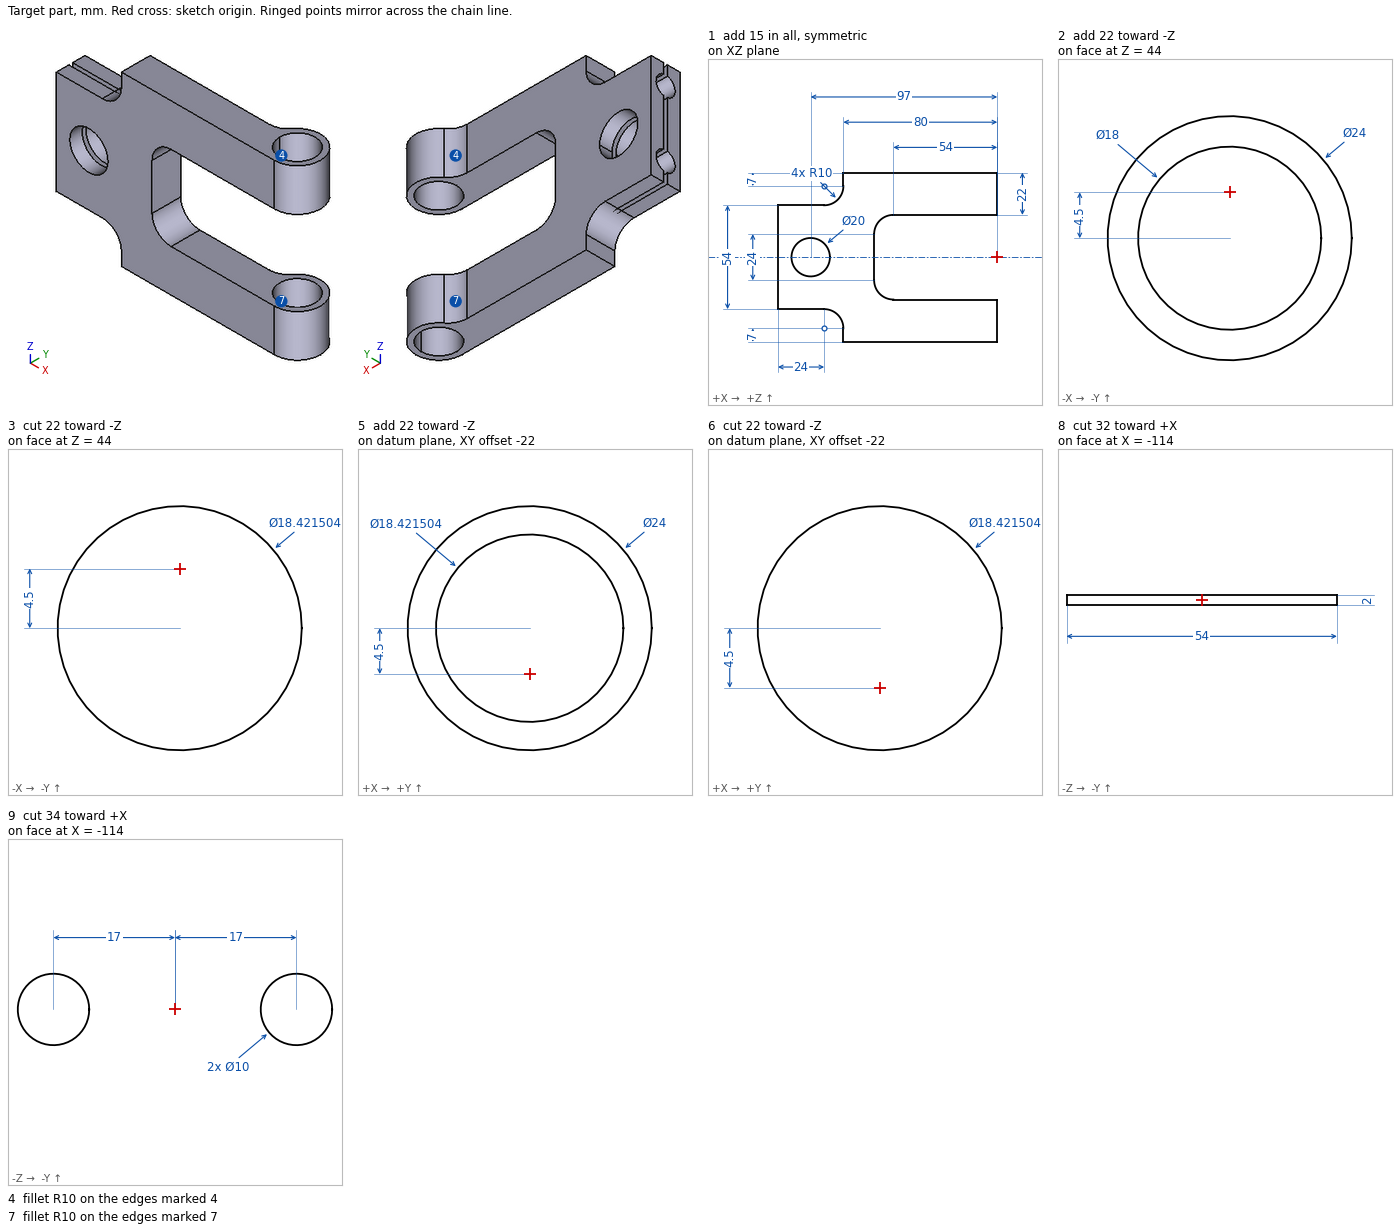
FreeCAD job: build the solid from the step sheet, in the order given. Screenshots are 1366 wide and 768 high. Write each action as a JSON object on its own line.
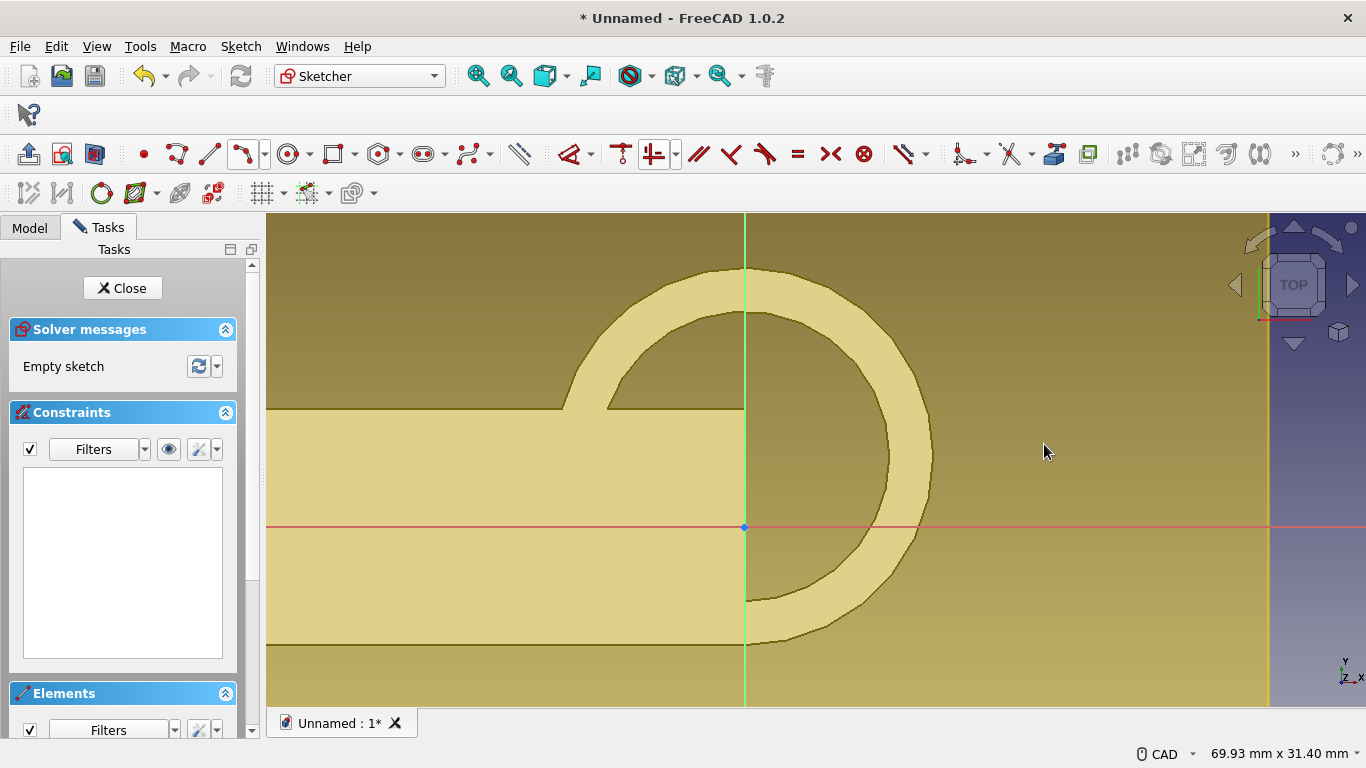
{"action": "left_click", "coordinate": [288, 154]}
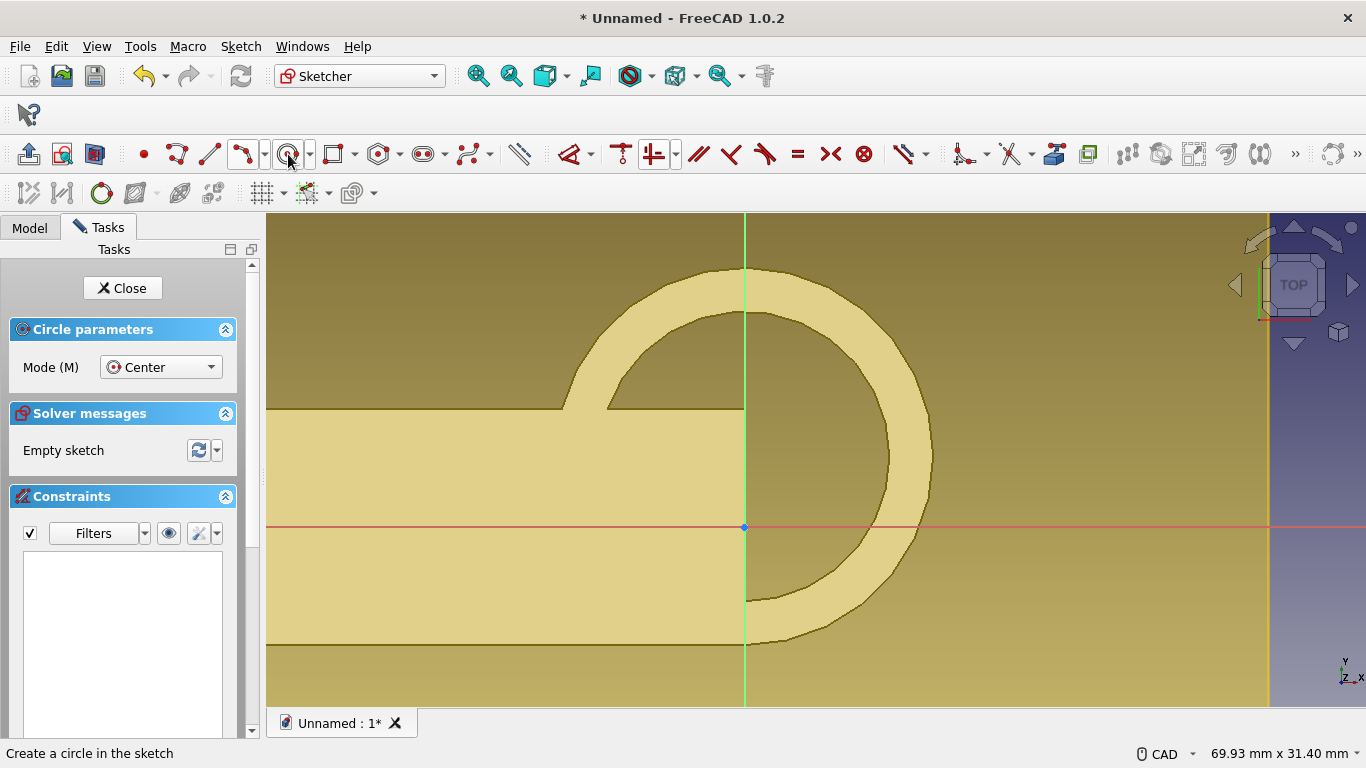
{"action": "left_click", "coordinate": [745, 456]}
{"action": "left_click", "coordinate": [847, 354]}
{"action": "key", "text": "Escape"}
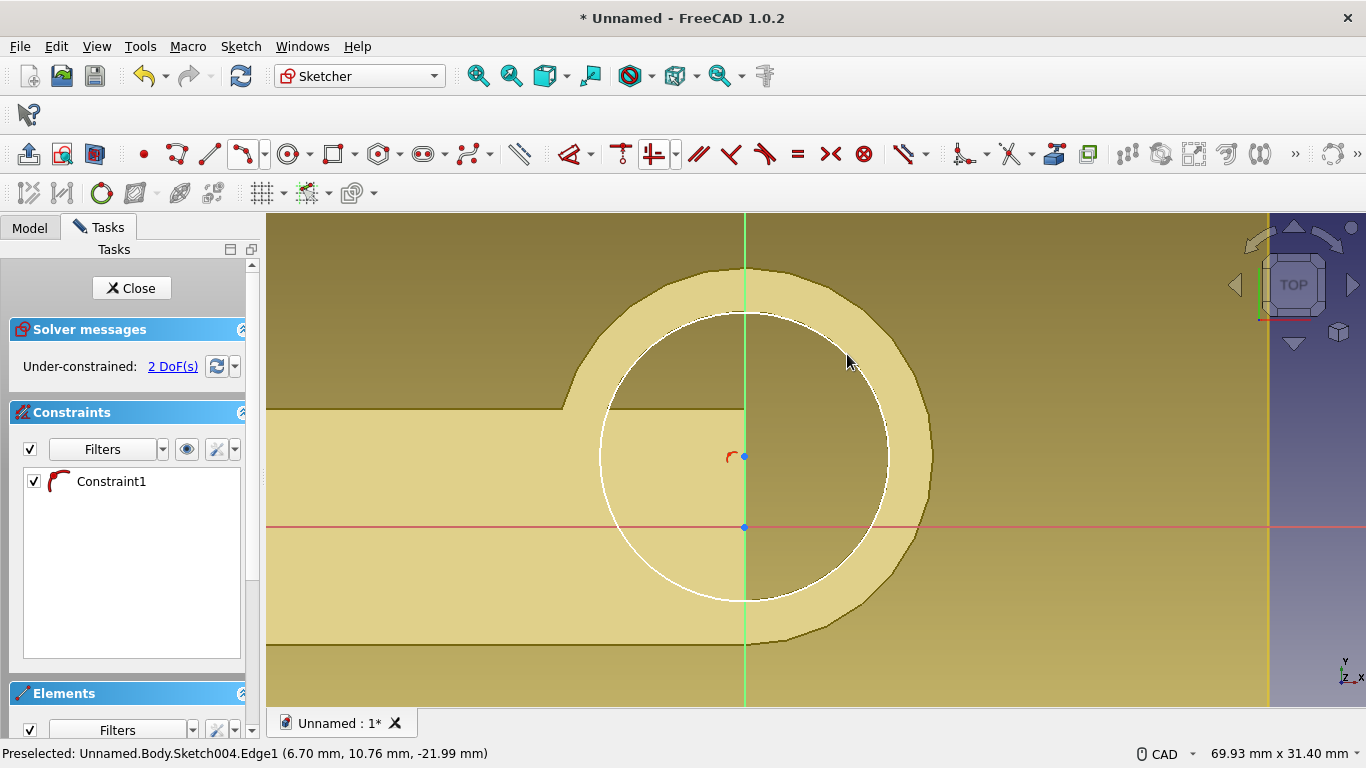
{"action": "left_click", "coordinate": [568, 154]}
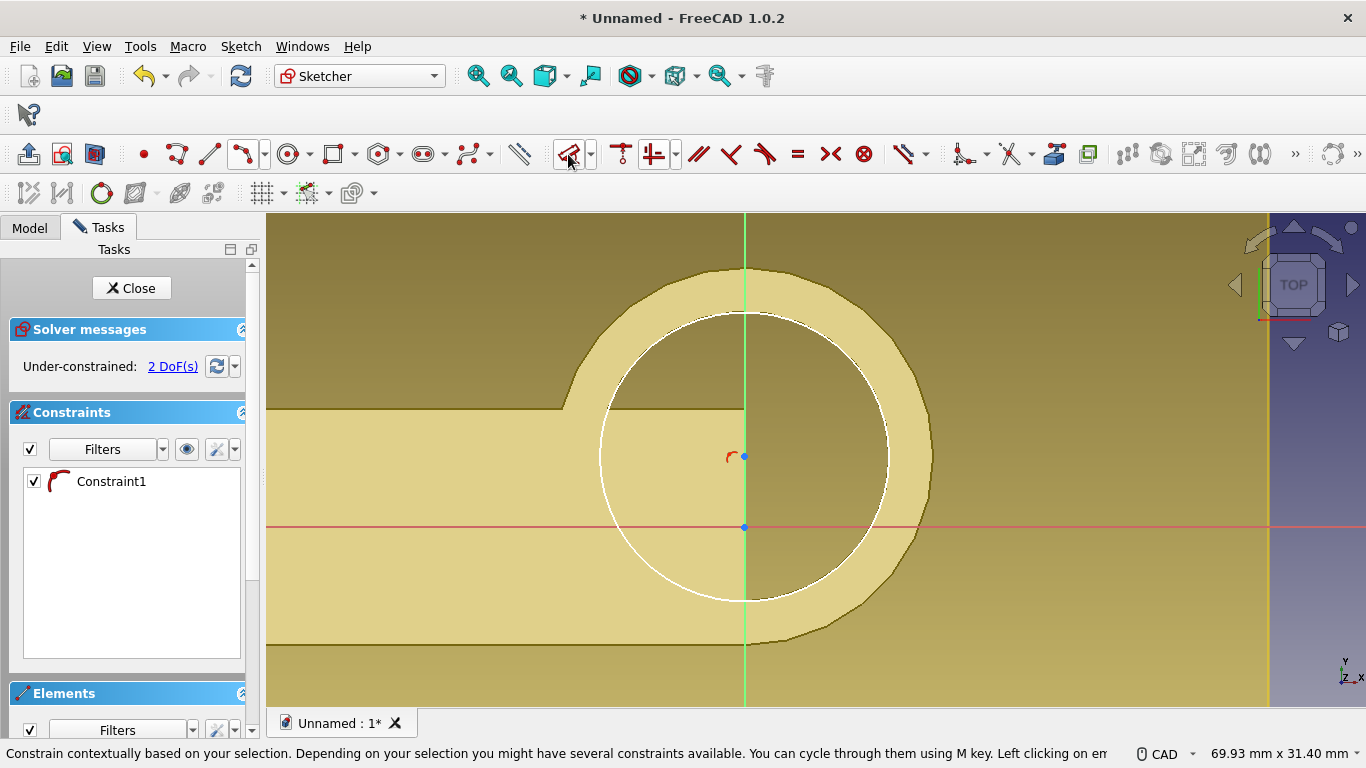
{"action": "left_click", "coordinate": [846, 354]}
{"action": "left_click", "coordinate": [868, 331]}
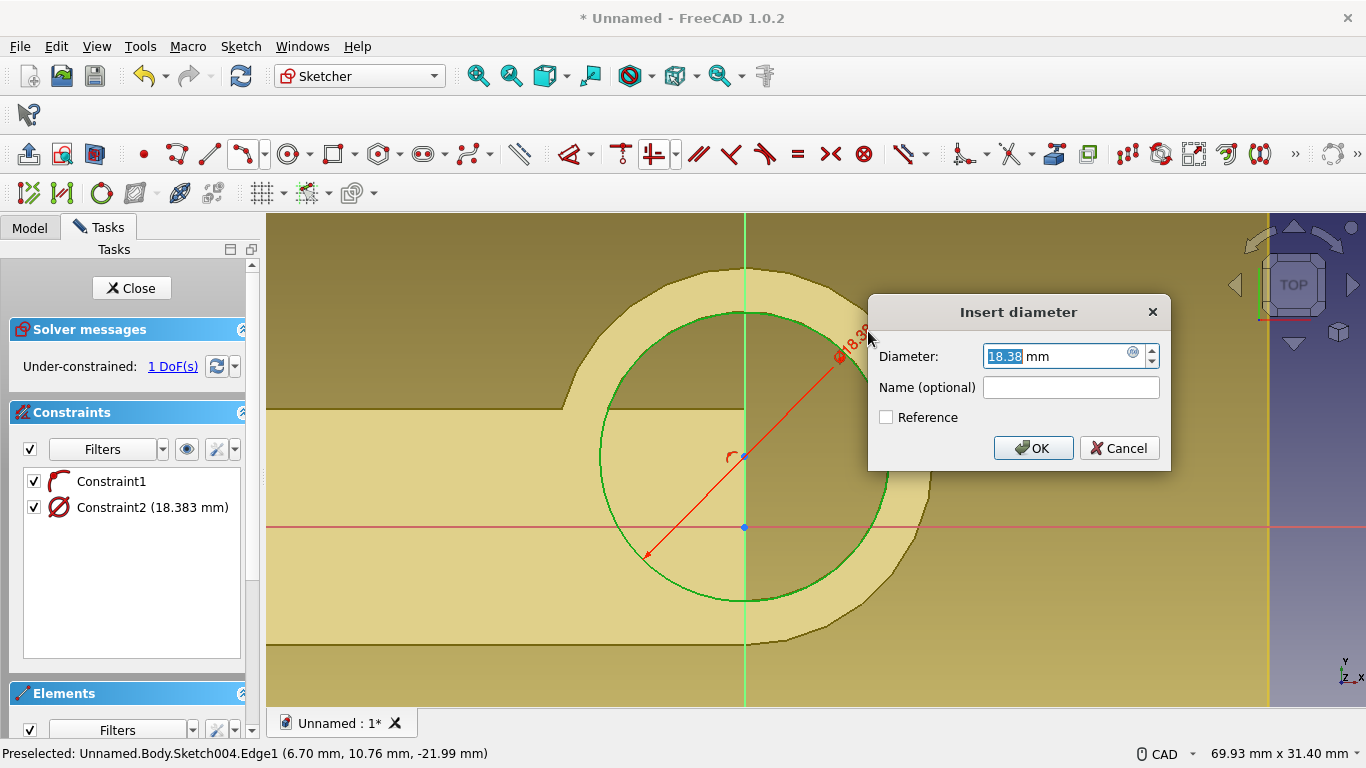
{"action": "type", "text": "18.421504"}
{"action": "key", "text": "Return"}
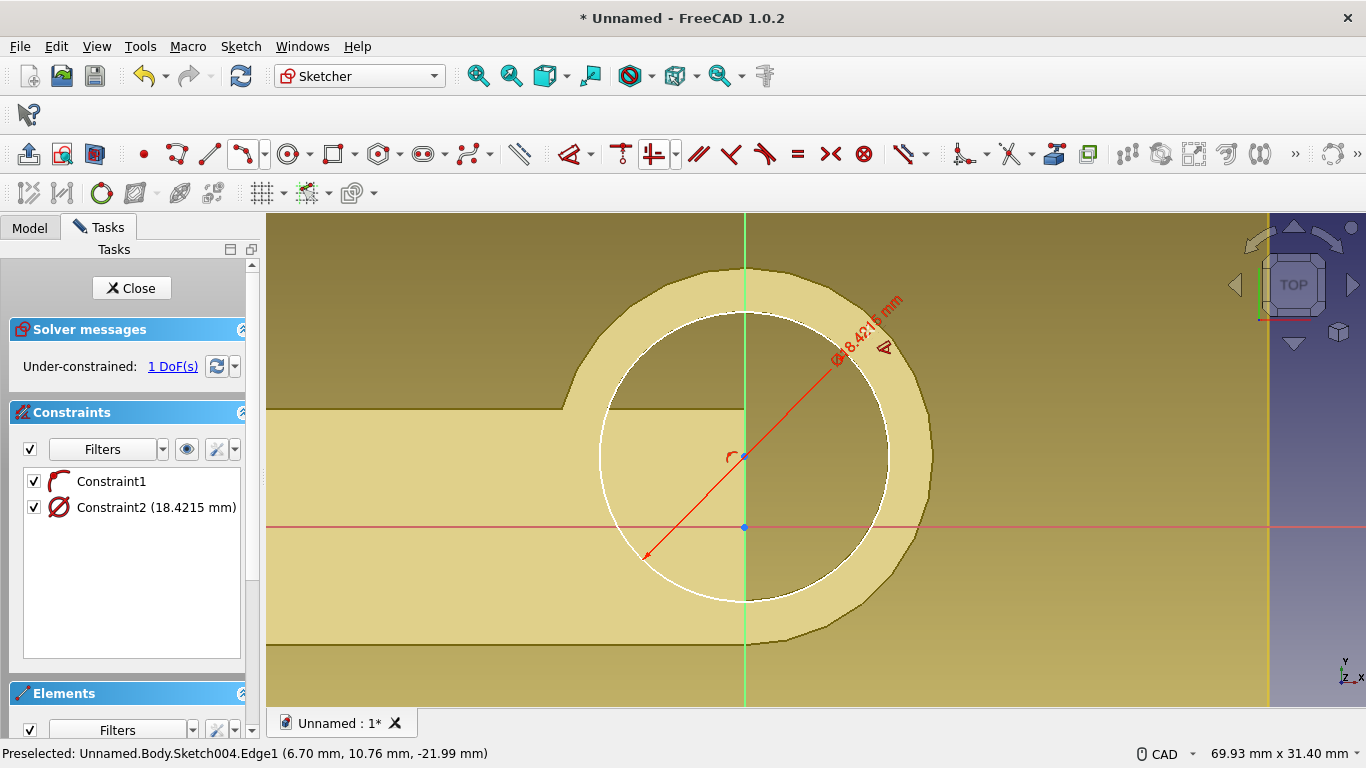
{"action": "left_click", "coordinate": [745, 457]}
{"action": "left_click", "coordinate": [779, 492]}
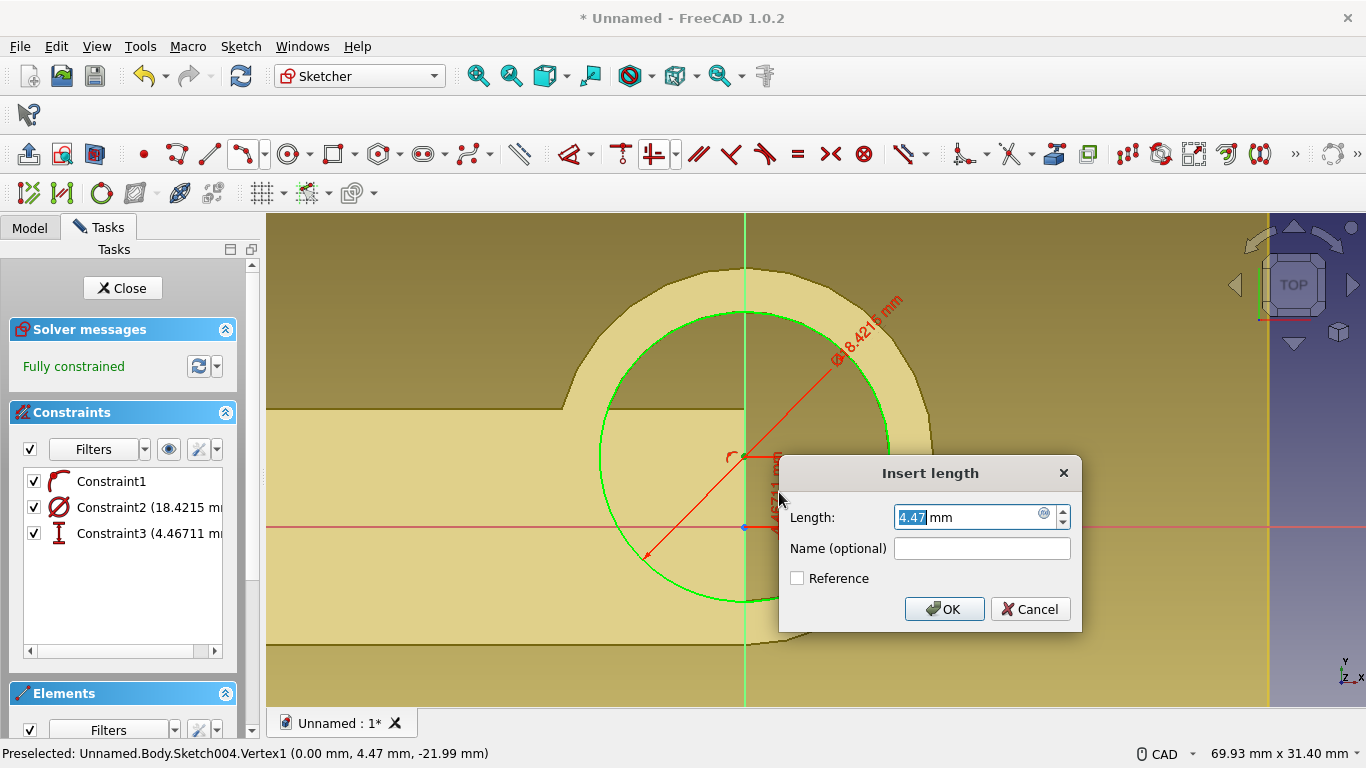
{"action": "type", "text": "4.5"}
{"action": "key", "text": "Return"}
{"action": "key", "text": "Escape"}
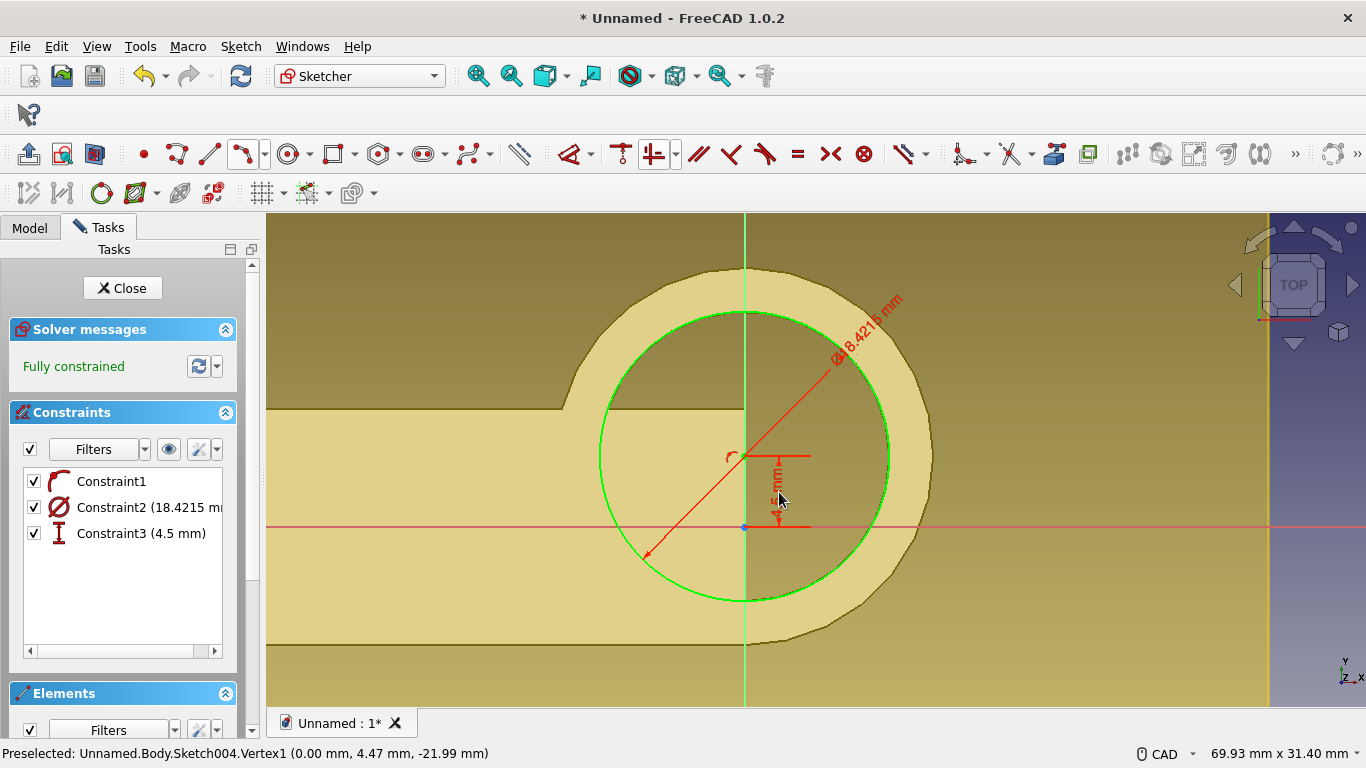
{"action": "left_click", "coordinate": [123, 288]}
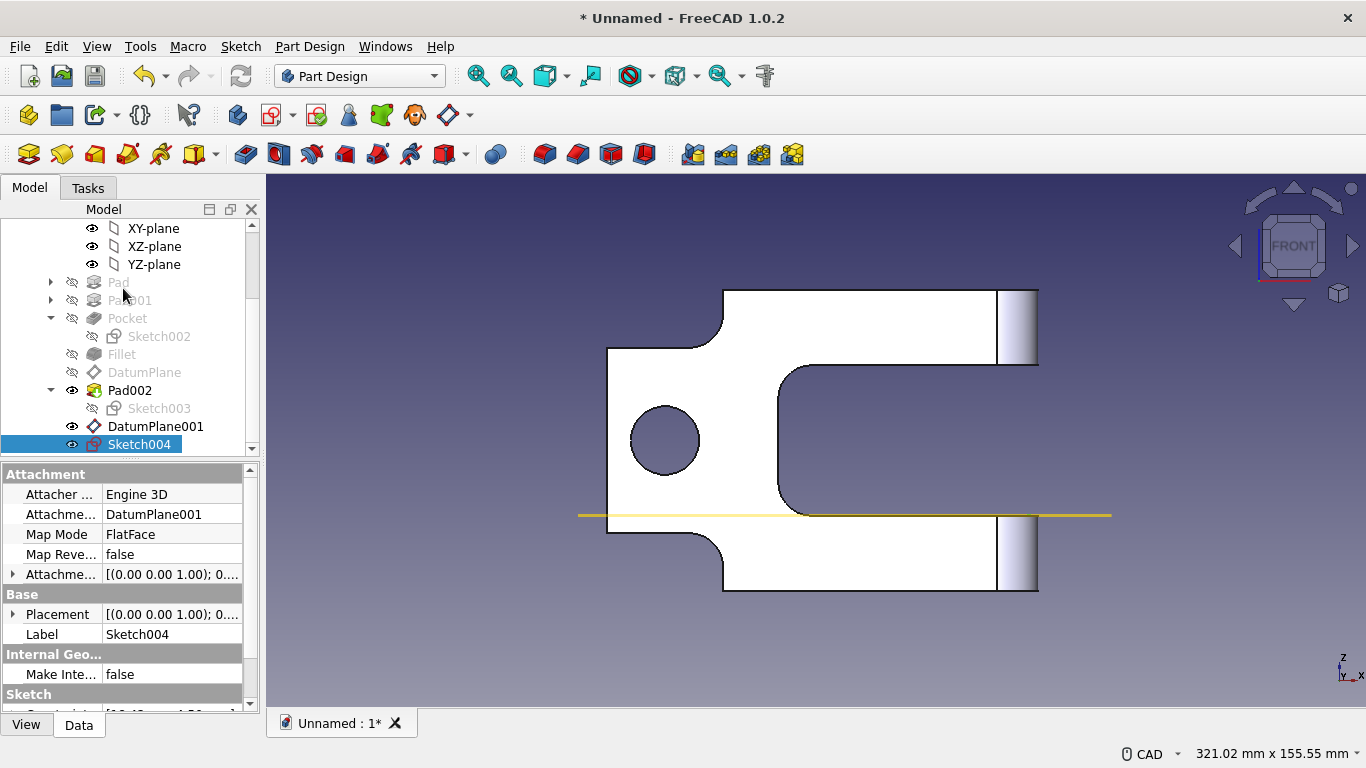
{"action": "left_click", "coordinate": [246, 154]}